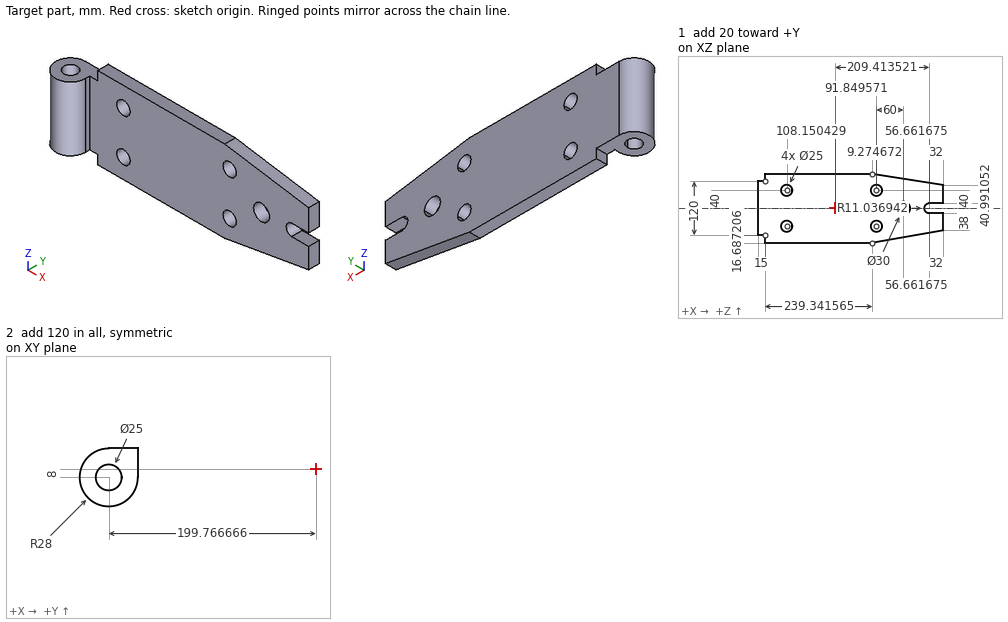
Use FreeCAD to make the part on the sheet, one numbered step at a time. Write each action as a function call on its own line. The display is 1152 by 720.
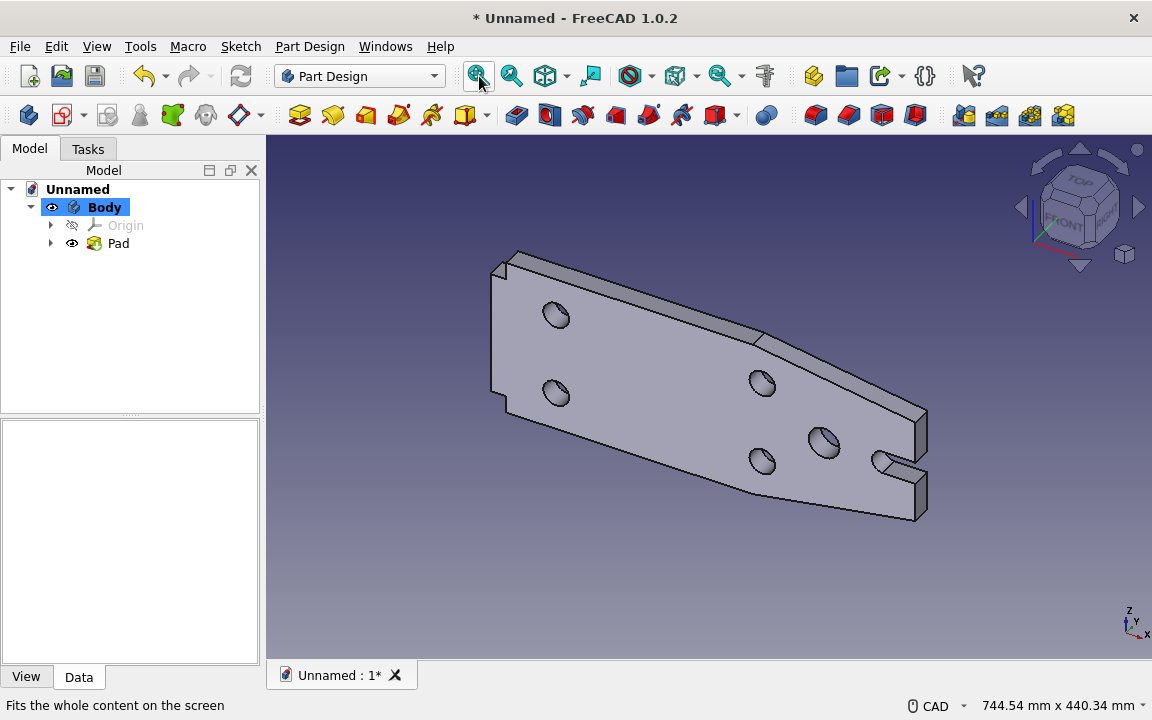
click(62, 116)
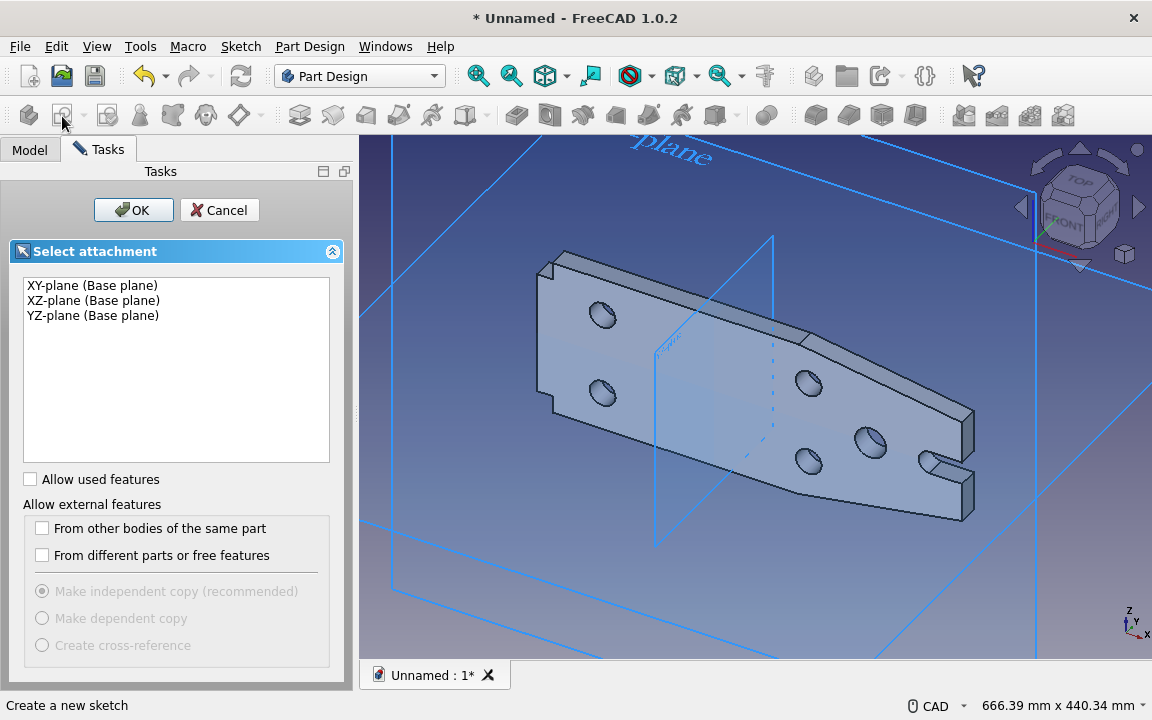
click(84, 286)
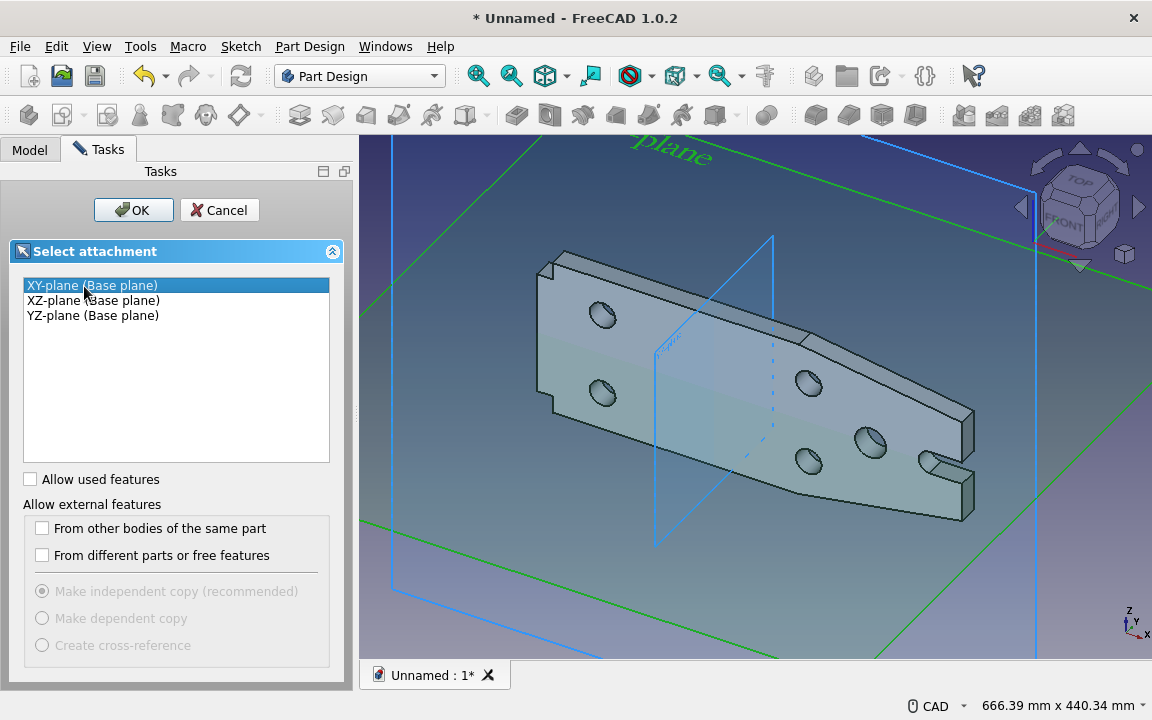
click(134, 210)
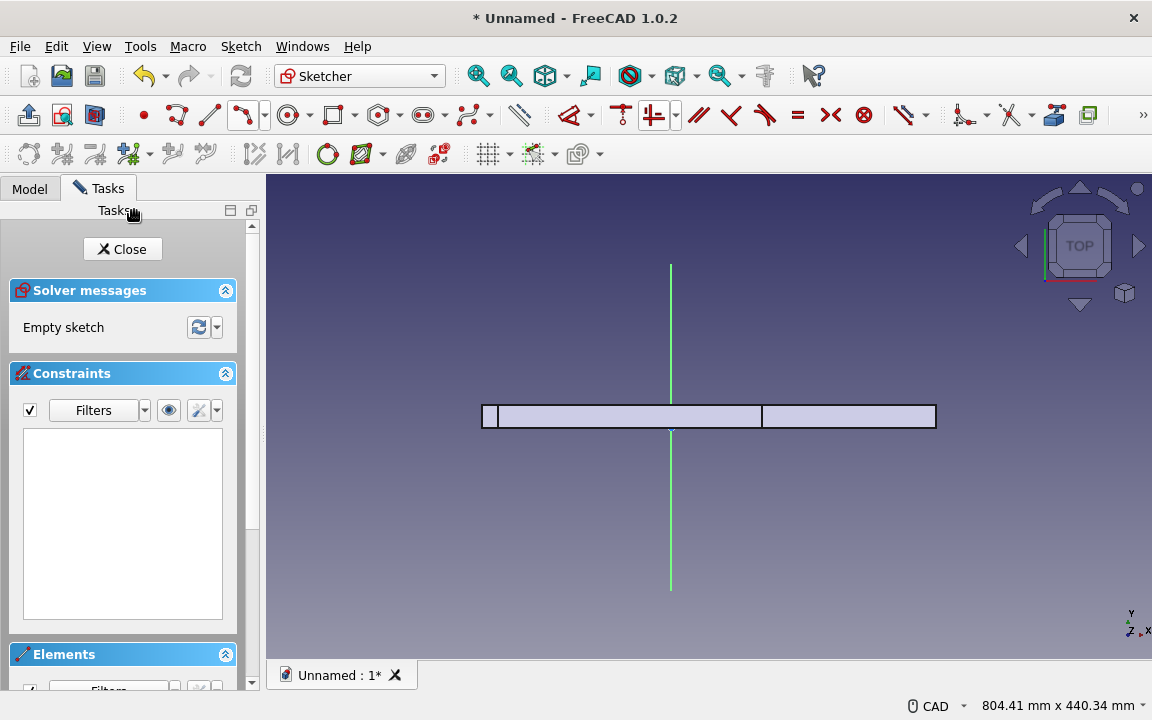
click(95, 116)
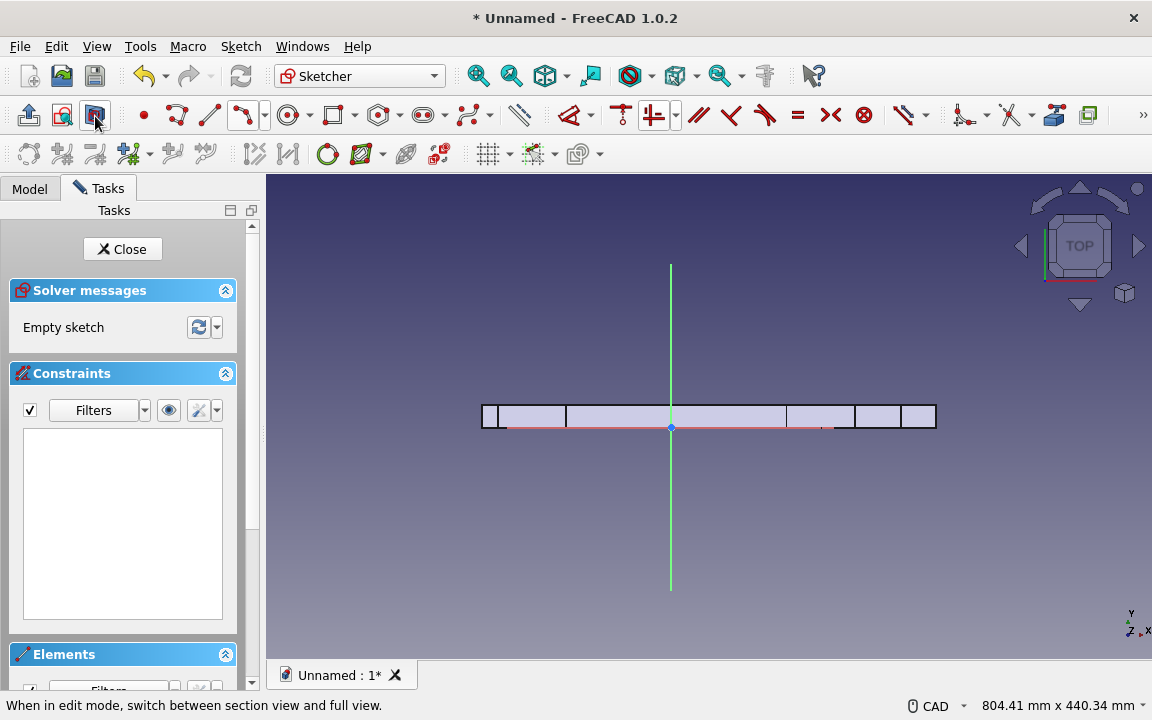
scroll(419, 435, up, 9)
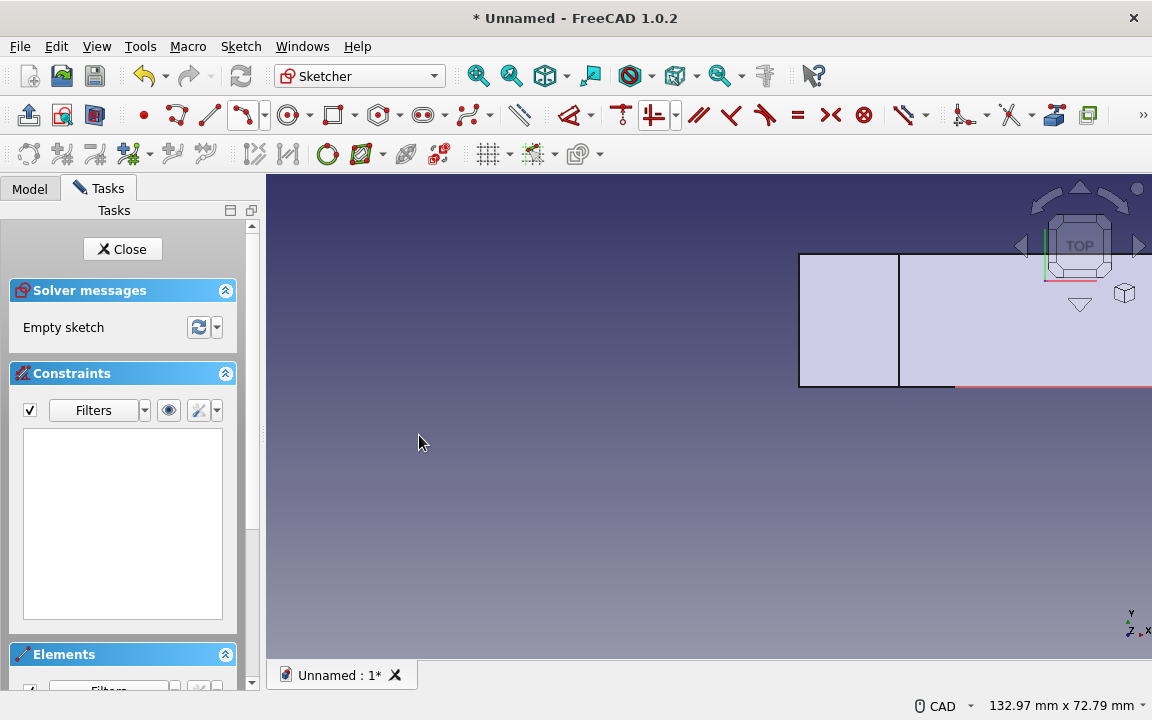
click(177, 116)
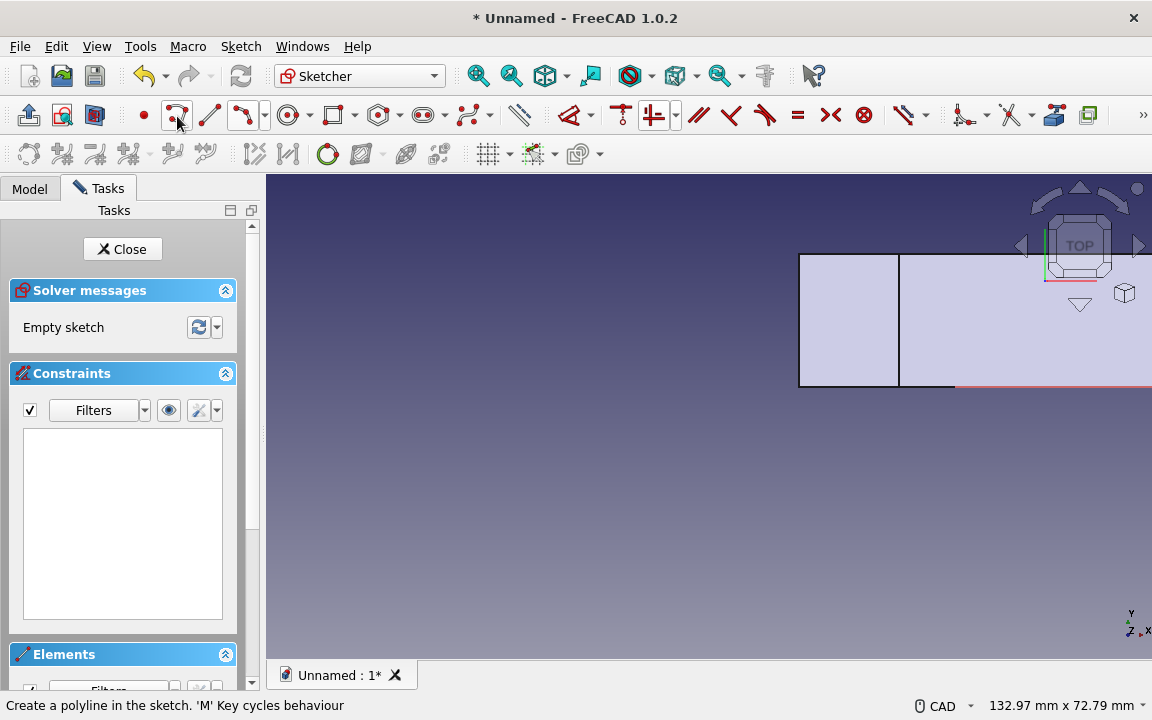
click(799, 440)
click(799, 254)
click(612, 254)
right_click(612, 254)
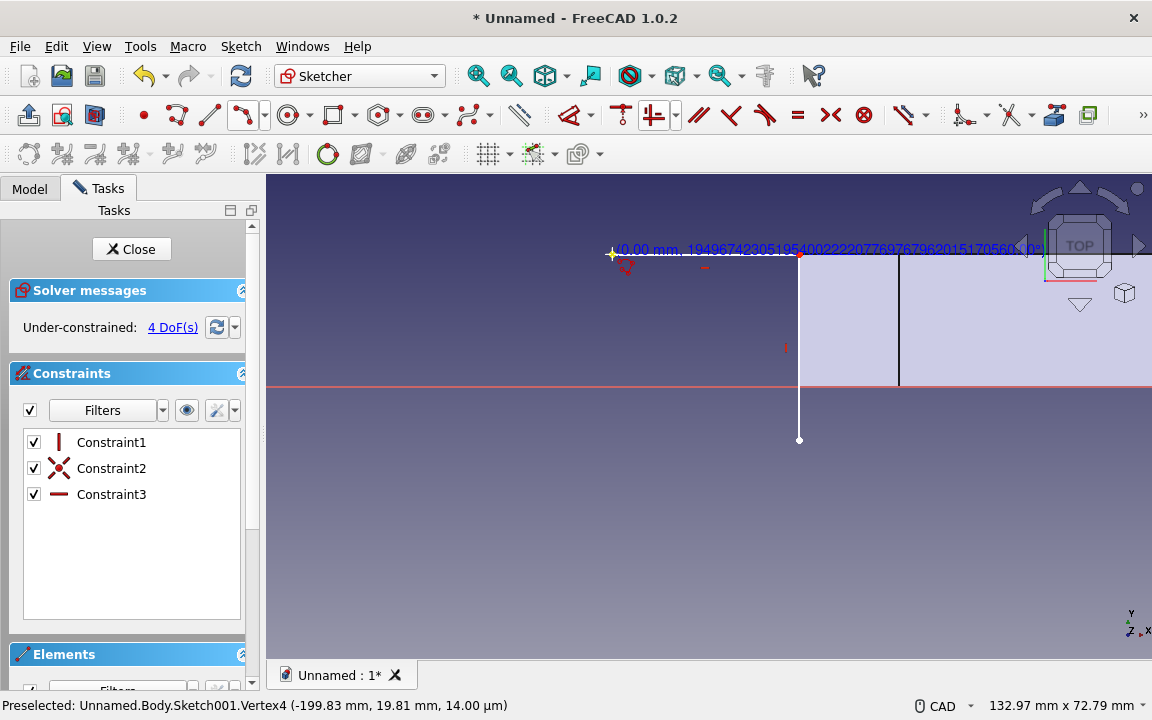
click(242, 116)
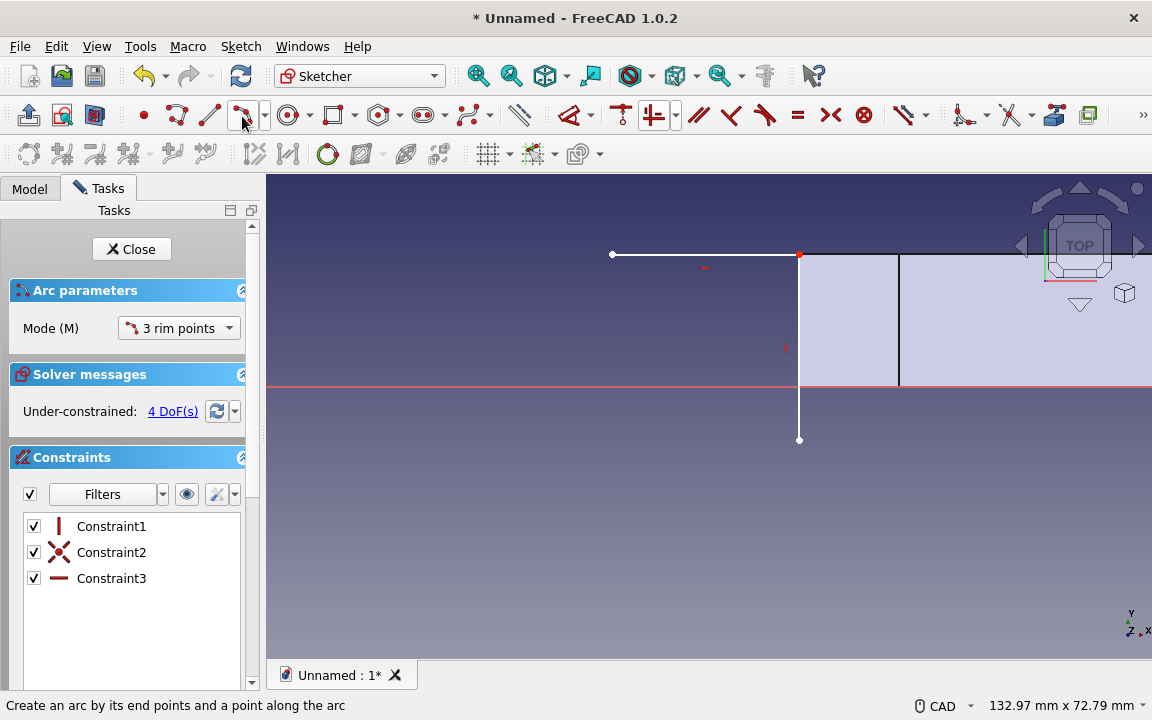
click(612, 255)
click(799, 441)
click(480, 572)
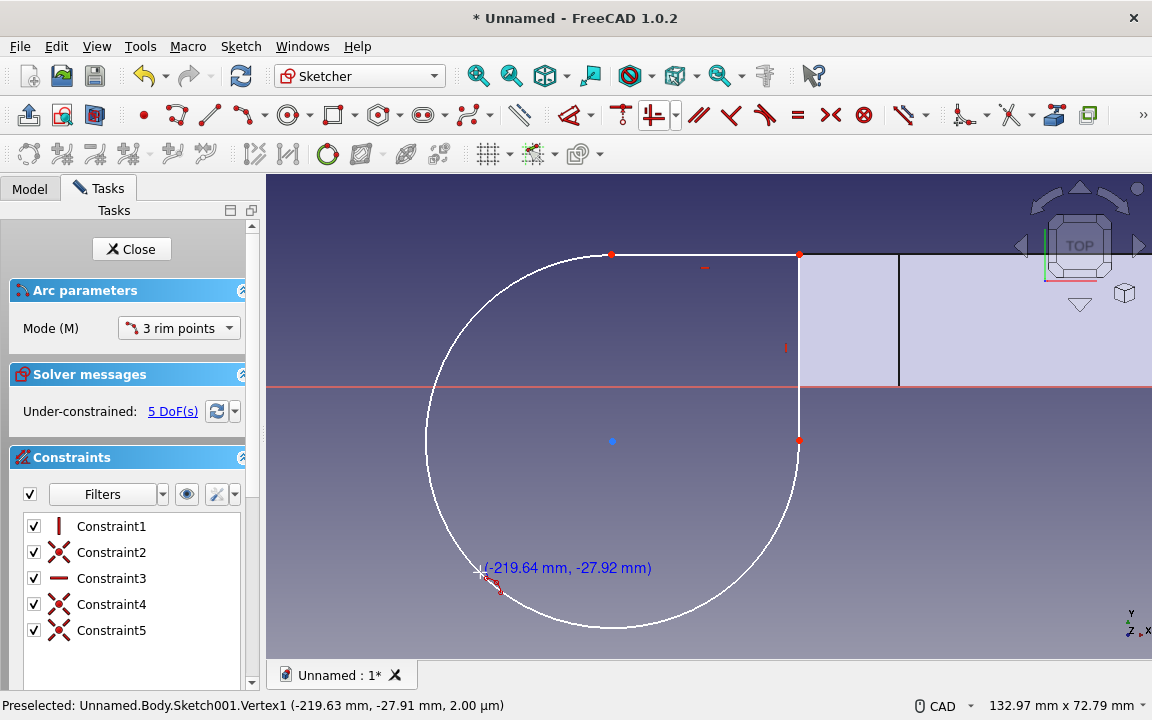
click(288, 116)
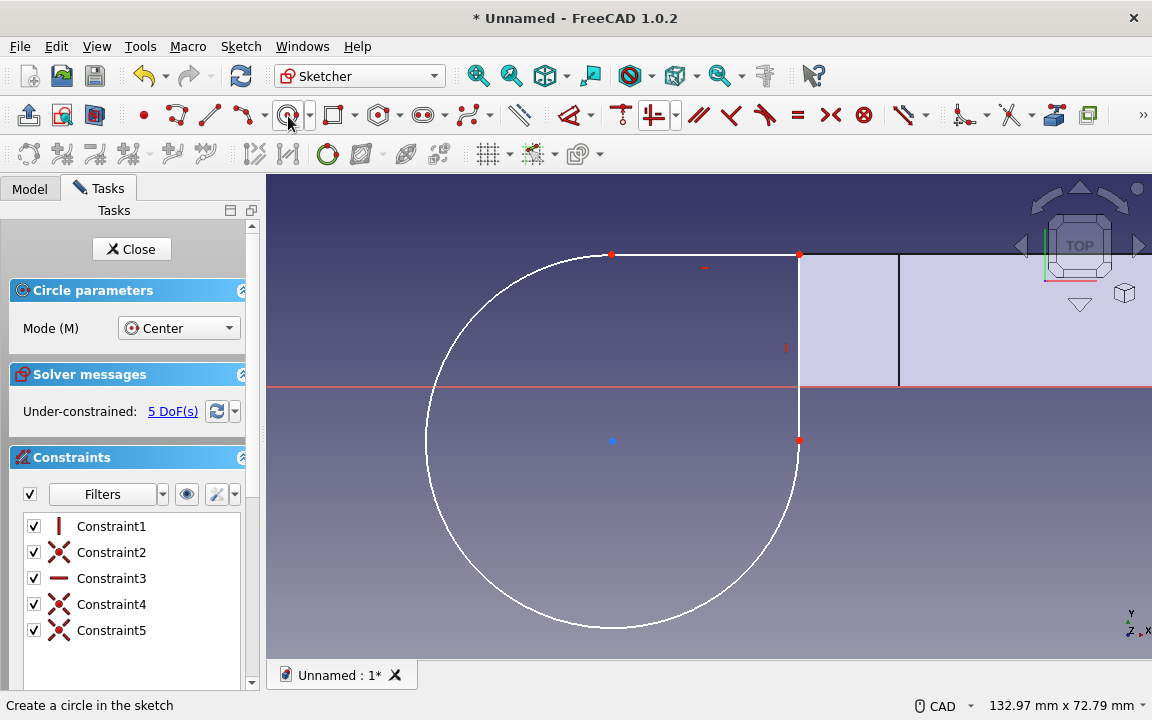
click(612, 440)
click(671, 499)
key(Escape)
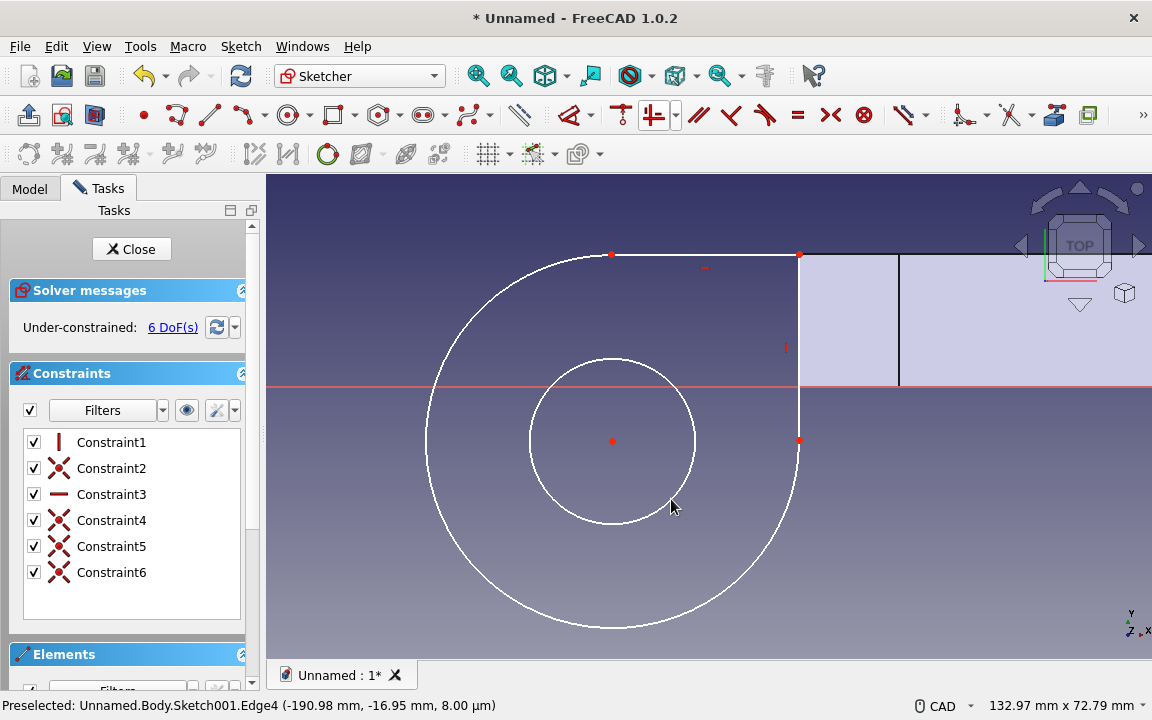
click(799, 385)